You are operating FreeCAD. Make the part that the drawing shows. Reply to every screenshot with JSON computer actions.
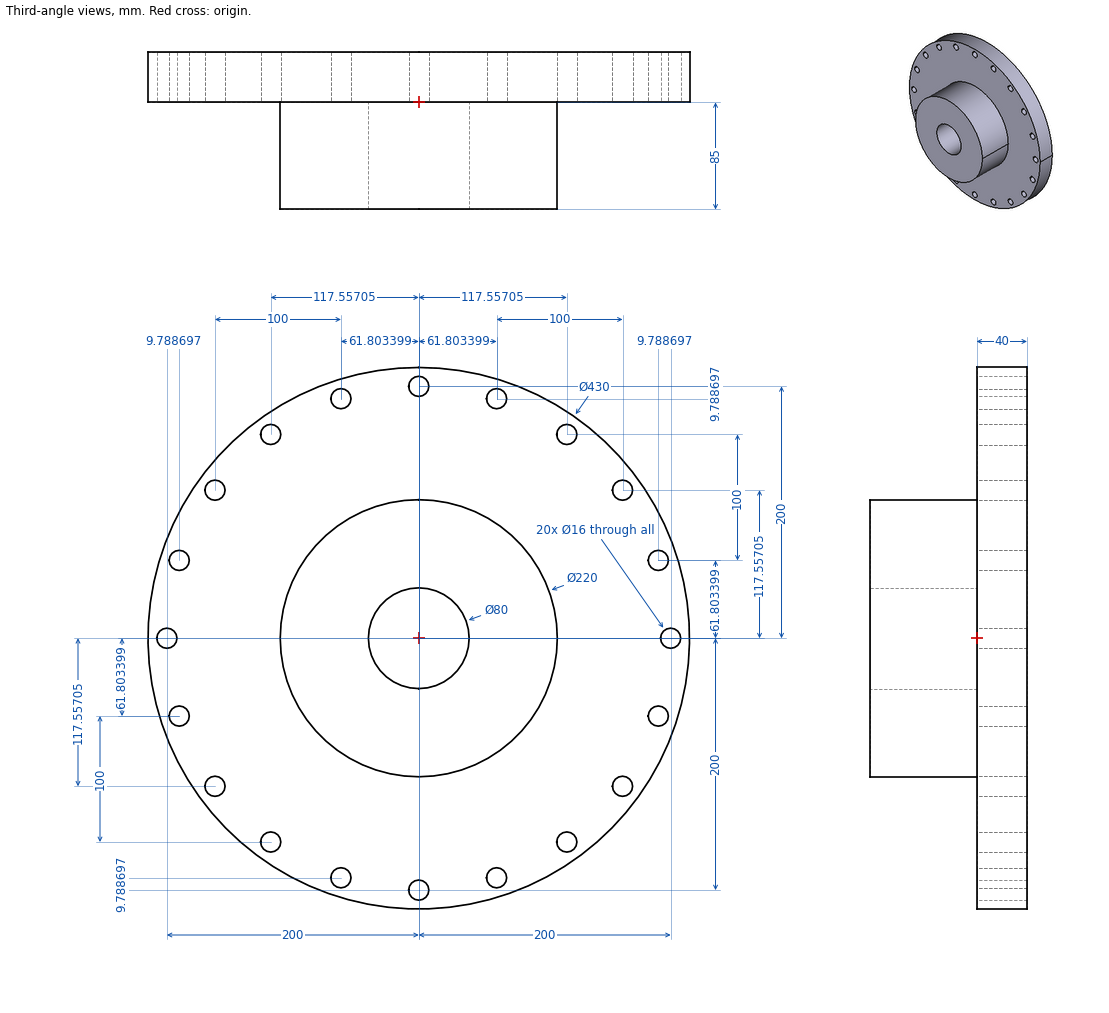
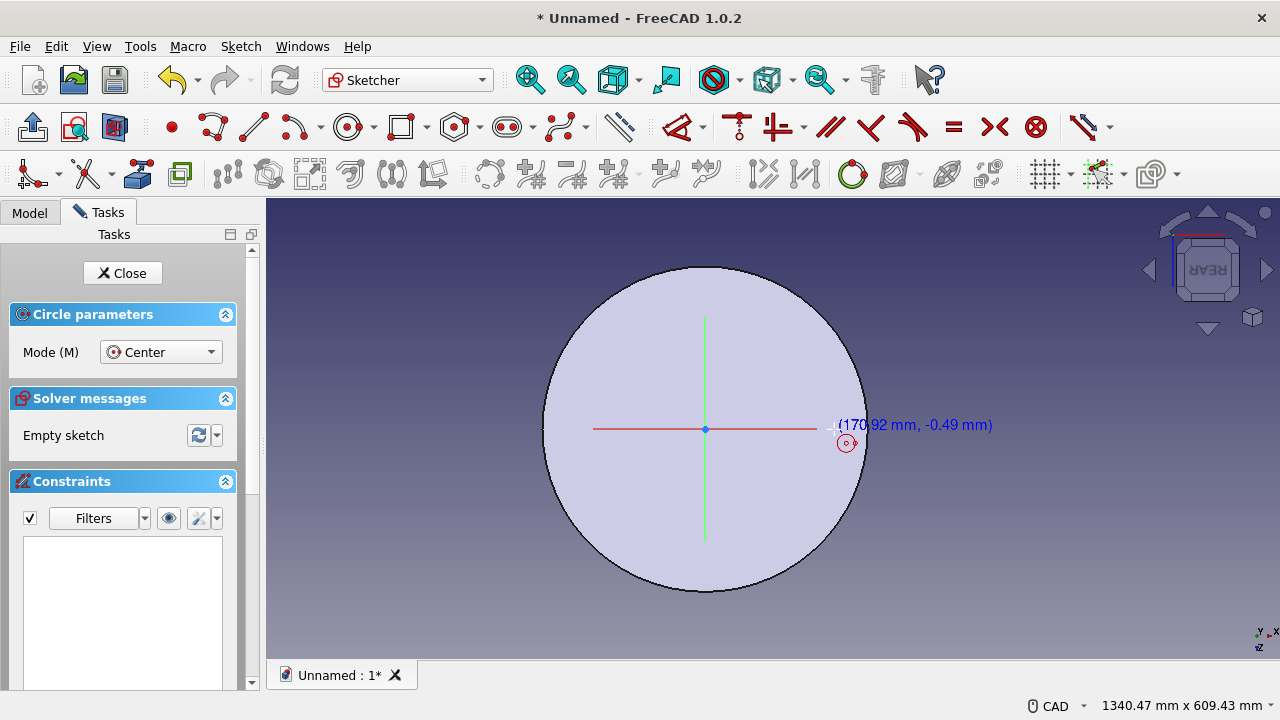
{"action": "left_click", "coordinate": [856, 429]}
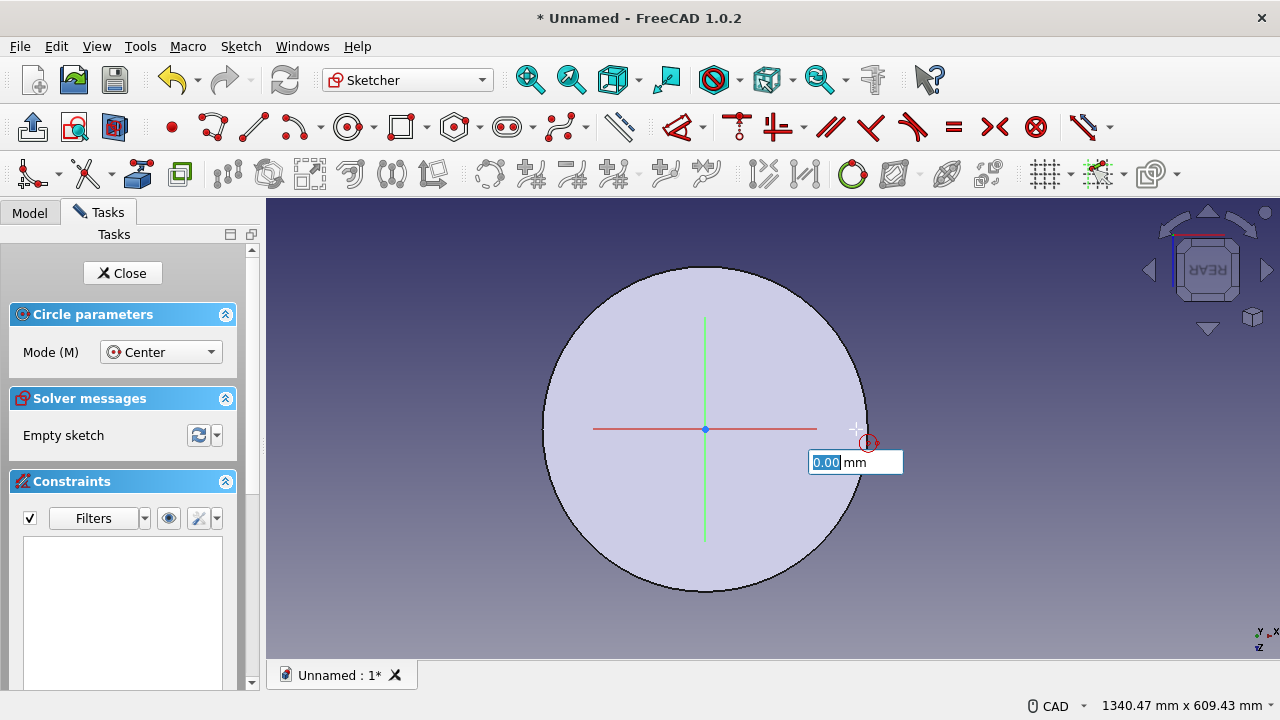
{"action": "scroll", "coordinate": [854, 435], "scroll_direction": "up", "scroll_amount": 6}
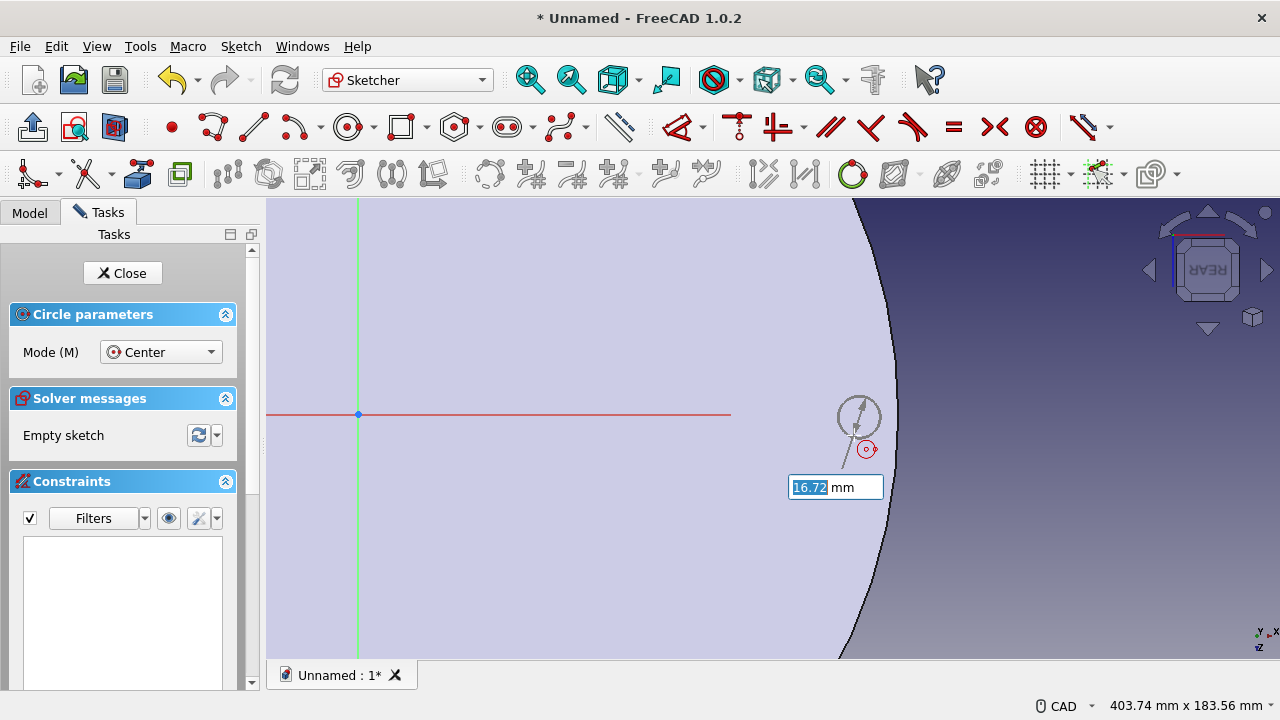
{"action": "left_click", "coordinate": [854, 434]}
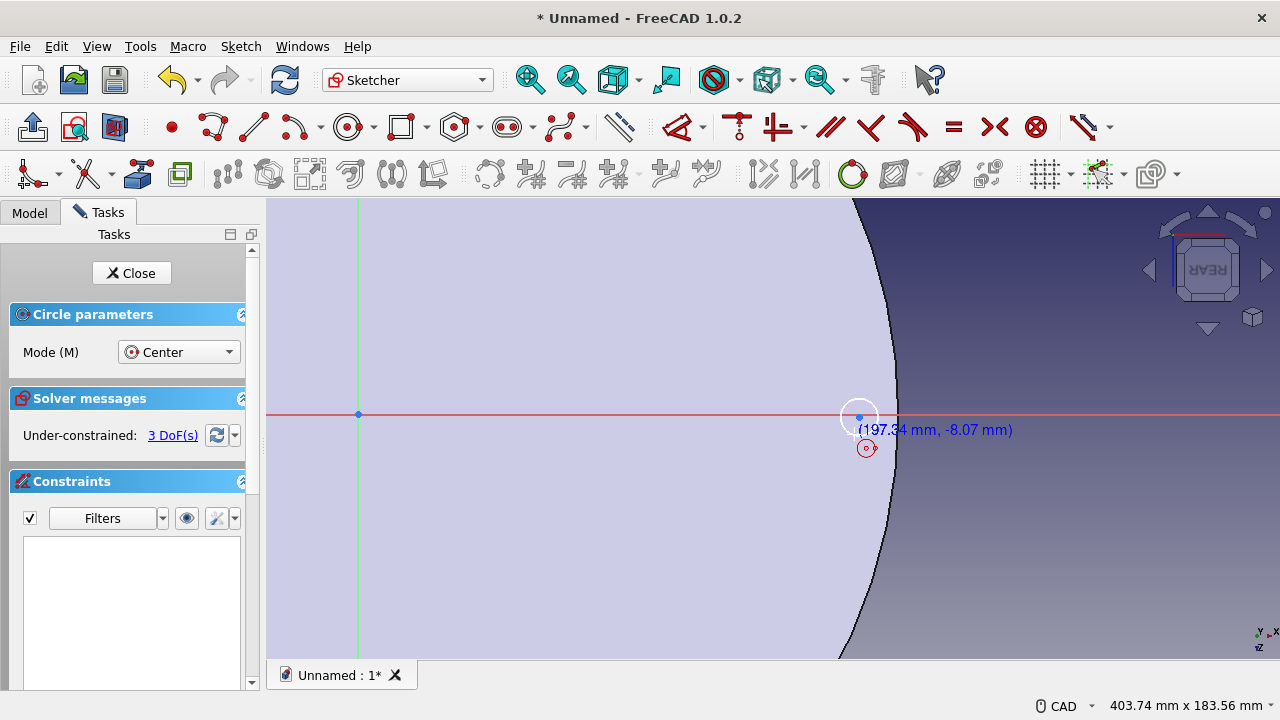
{"action": "left_click", "coordinate": [836, 570]}
{"action": "left_click", "coordinate": [850, 556]}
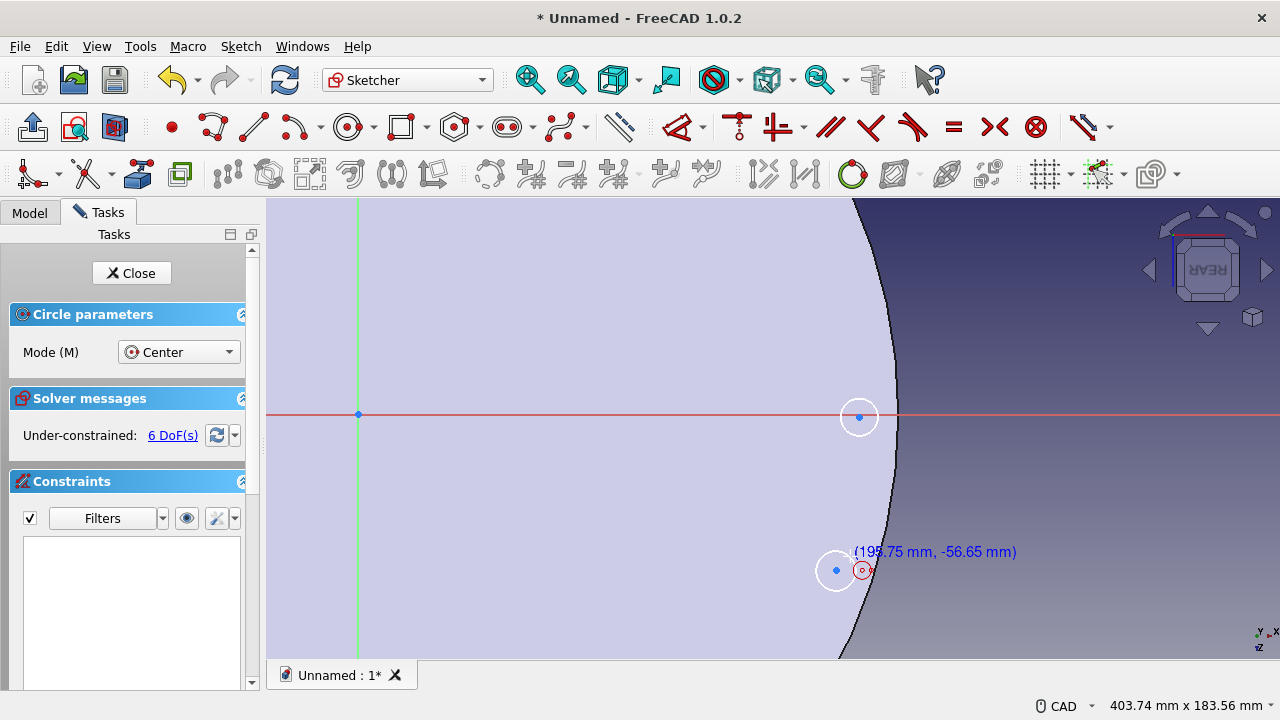
{"action": "scroll", "coordinate": [854, 434], "scroll_direction": "down", "scroll_amount": 6}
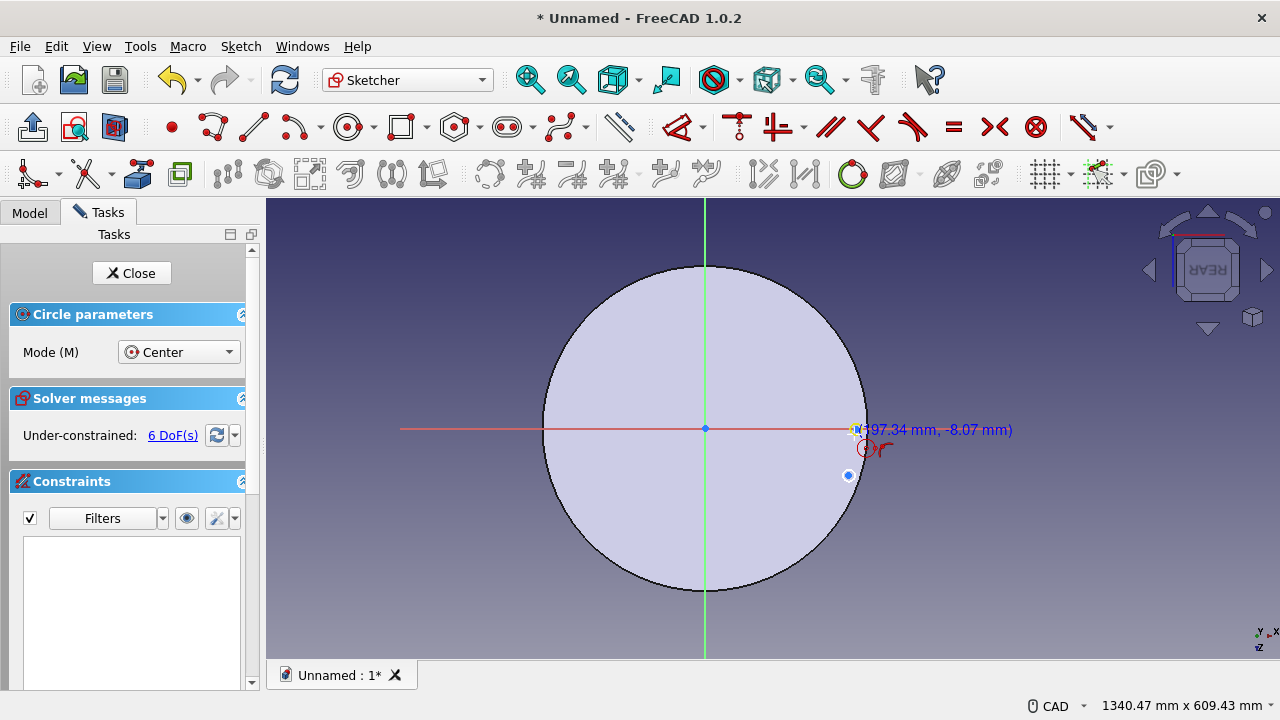
{"action": "scroll", "coordinate": [828, 517], "scroll_direction": "up", "scroll_amount": 7}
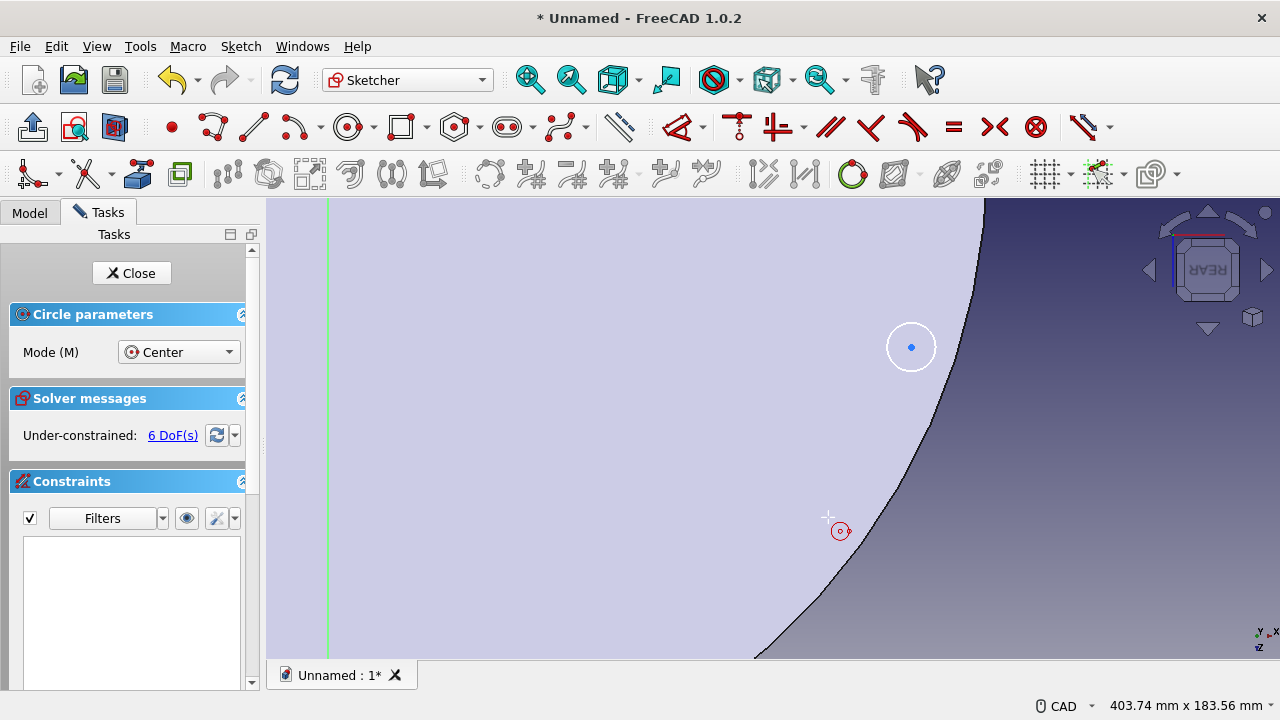
{"action": "scroll", "coordinate": [828, 518], "scroll_direction": "down", "scroll_amount": 7}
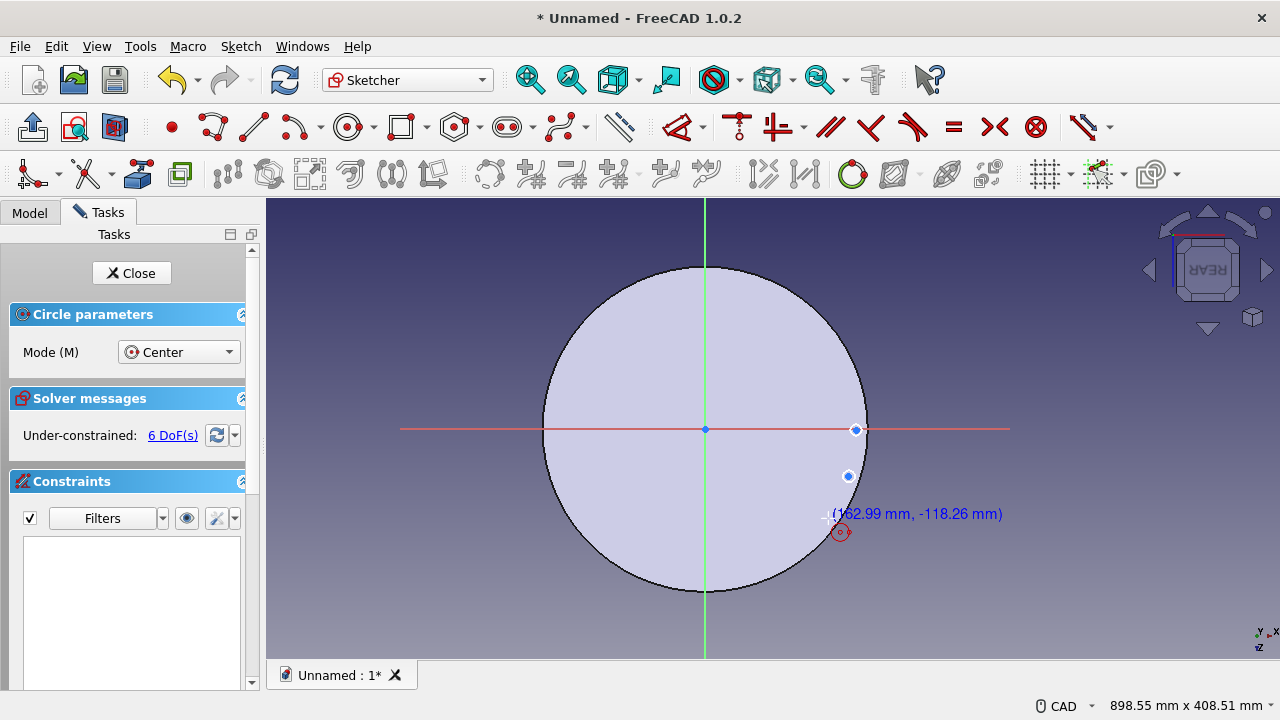
{"action": "left_click", "coordinate": [828, 518]}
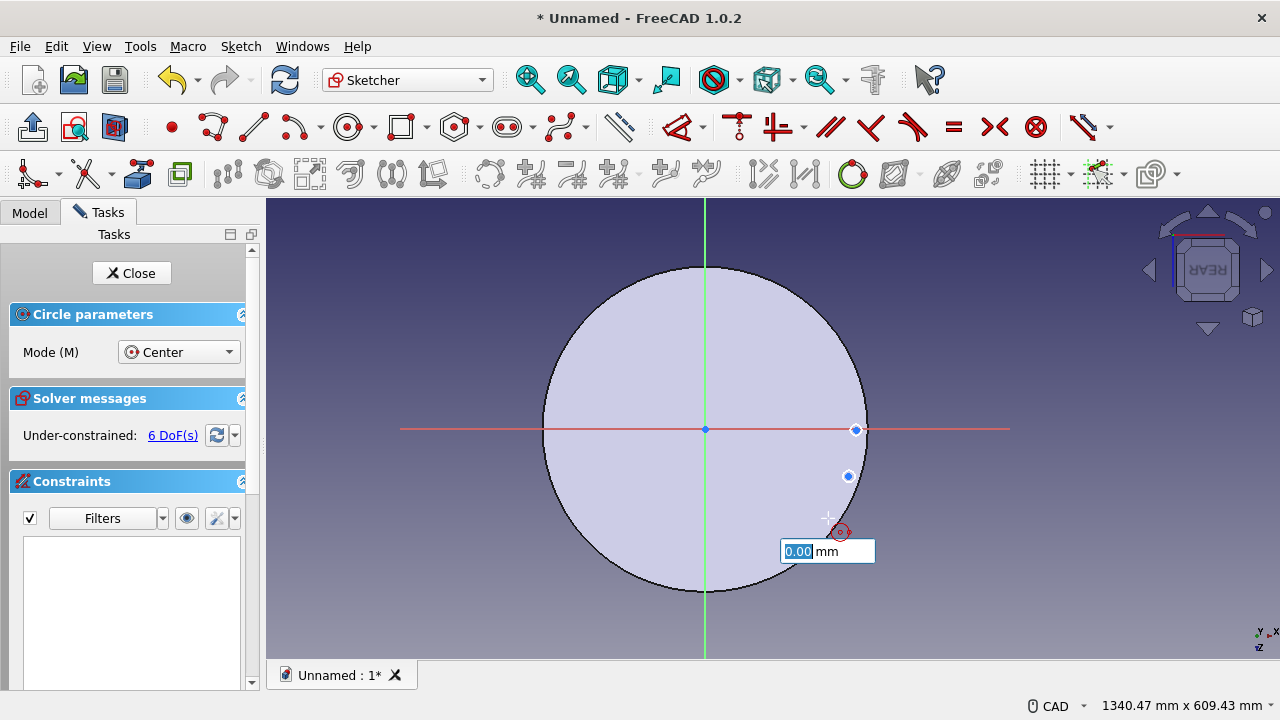
{"action": "scroll", "coordinate": [832, 514], "scroll_direction": "up", "scroll_amount": 5}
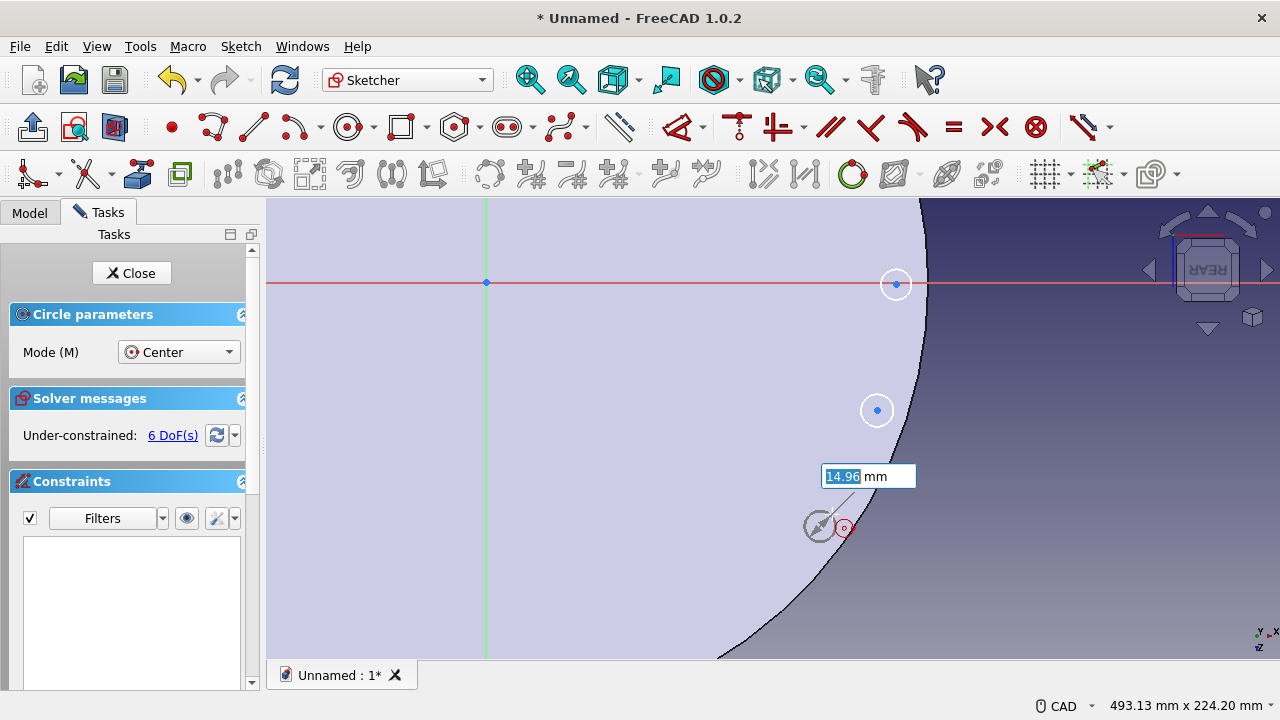
{"action": "left_click", "coordinate": [831, 513]}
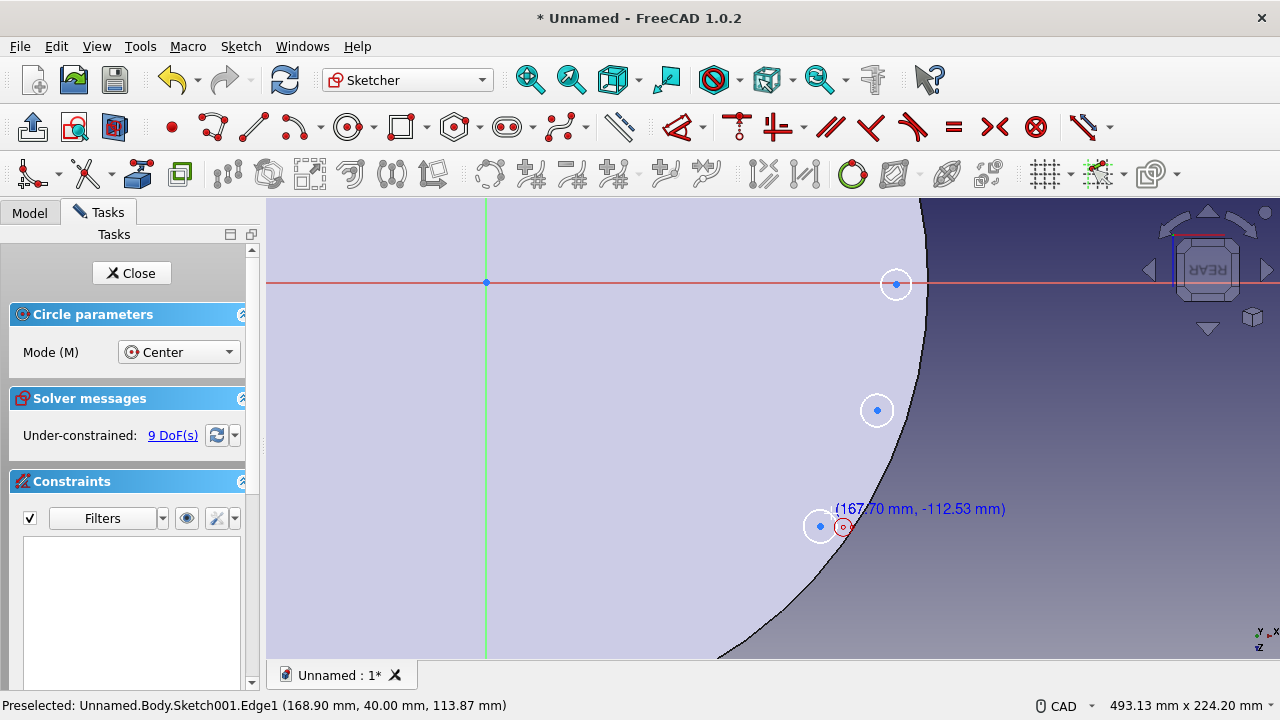
{"action": "scroll", "coordinate": [728, 615], "scroll_direction": "up", "scroll_amount": 2}